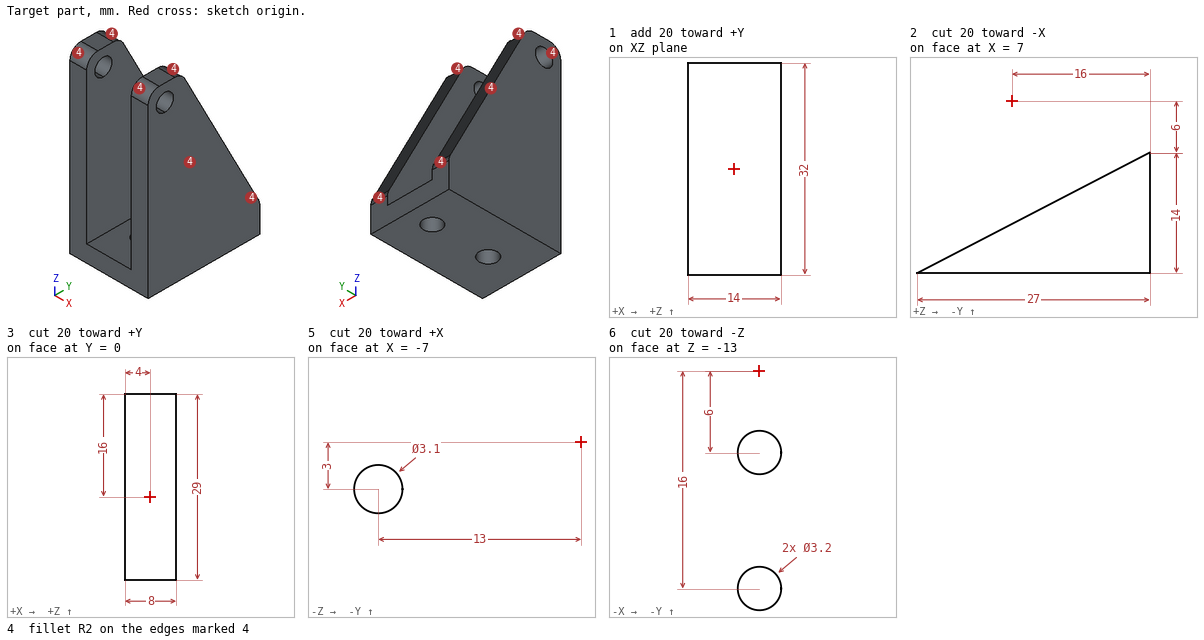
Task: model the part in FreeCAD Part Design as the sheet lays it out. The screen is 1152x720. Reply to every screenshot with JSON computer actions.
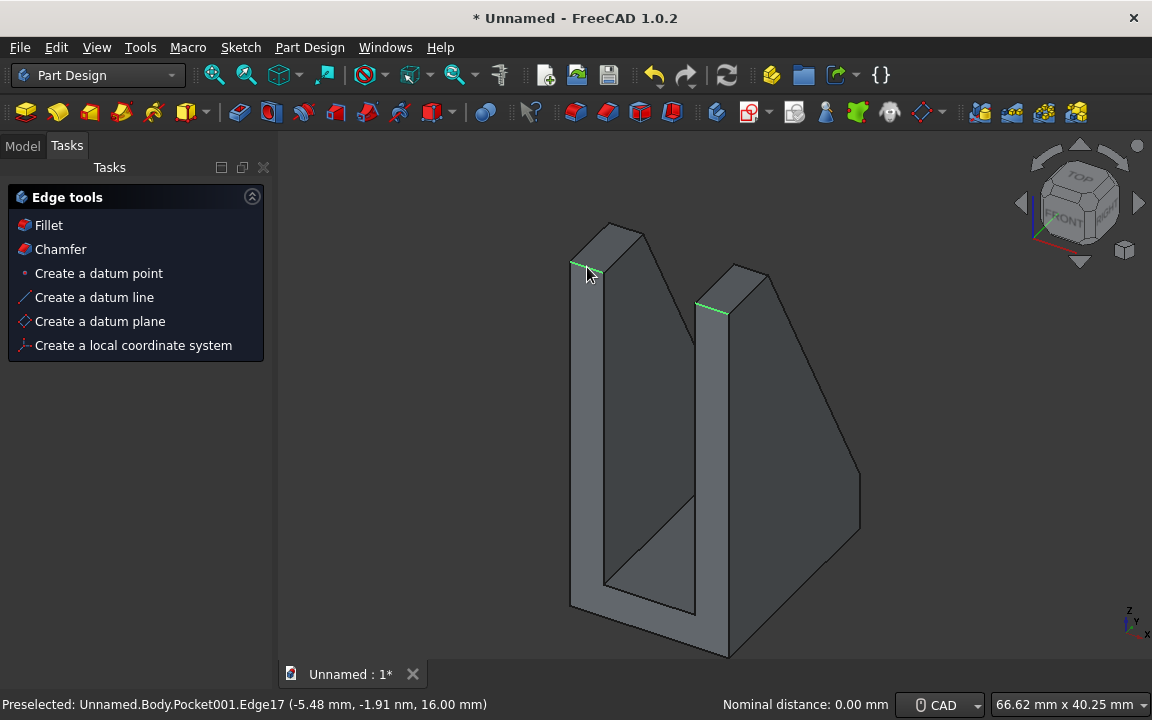
{"action": "key", "text": "0"}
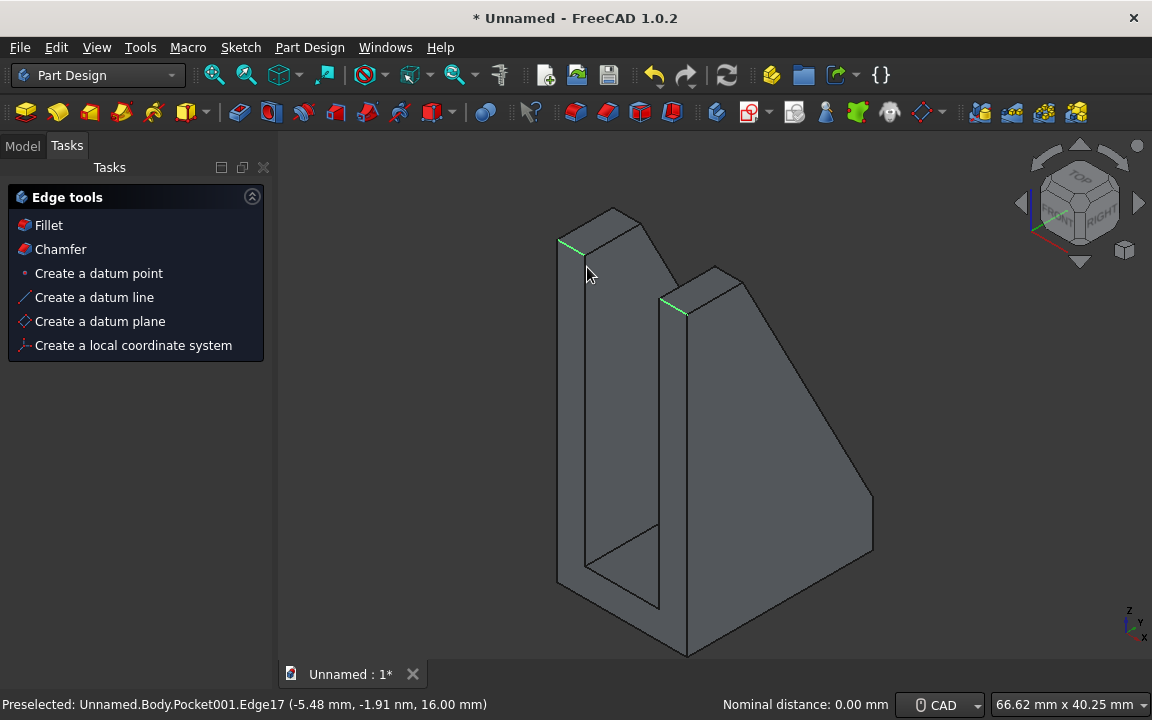
{"action": "key", "text": "2"}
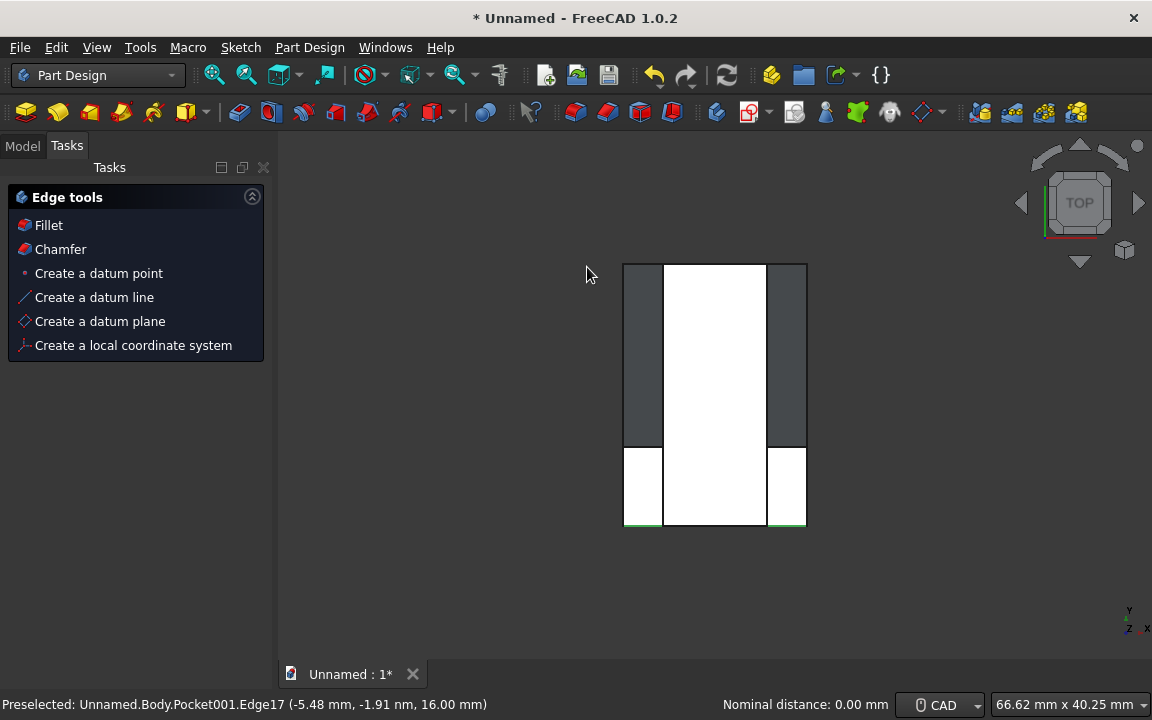
{"action": "left_click", "coordinate": [643, 446], "text": "ctrl"}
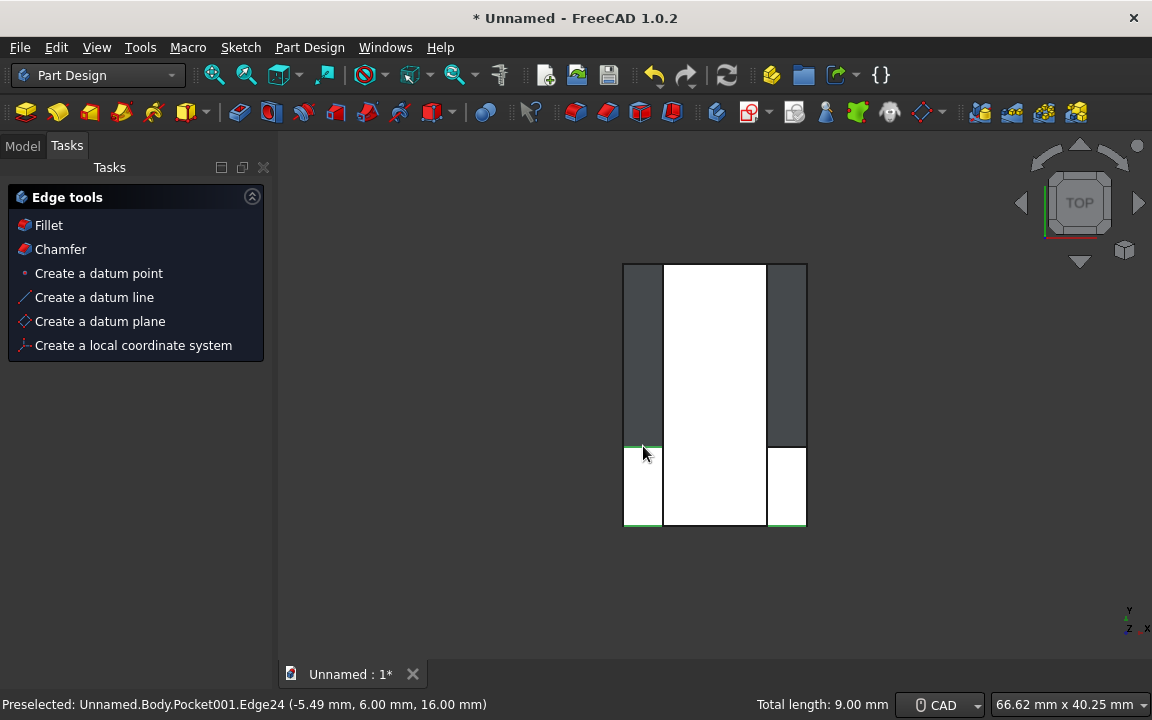
{"action": "left_click", "coordinate": [787, 446], "text": "ctrl"}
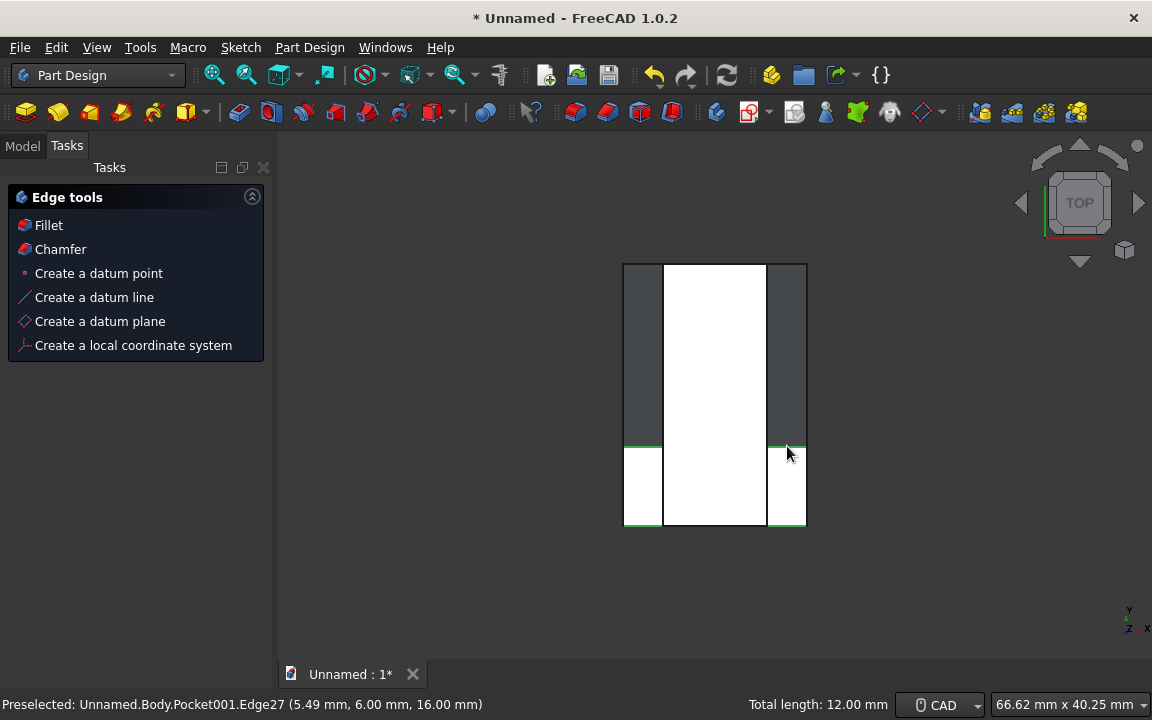
{"action": "key", "text": "1"}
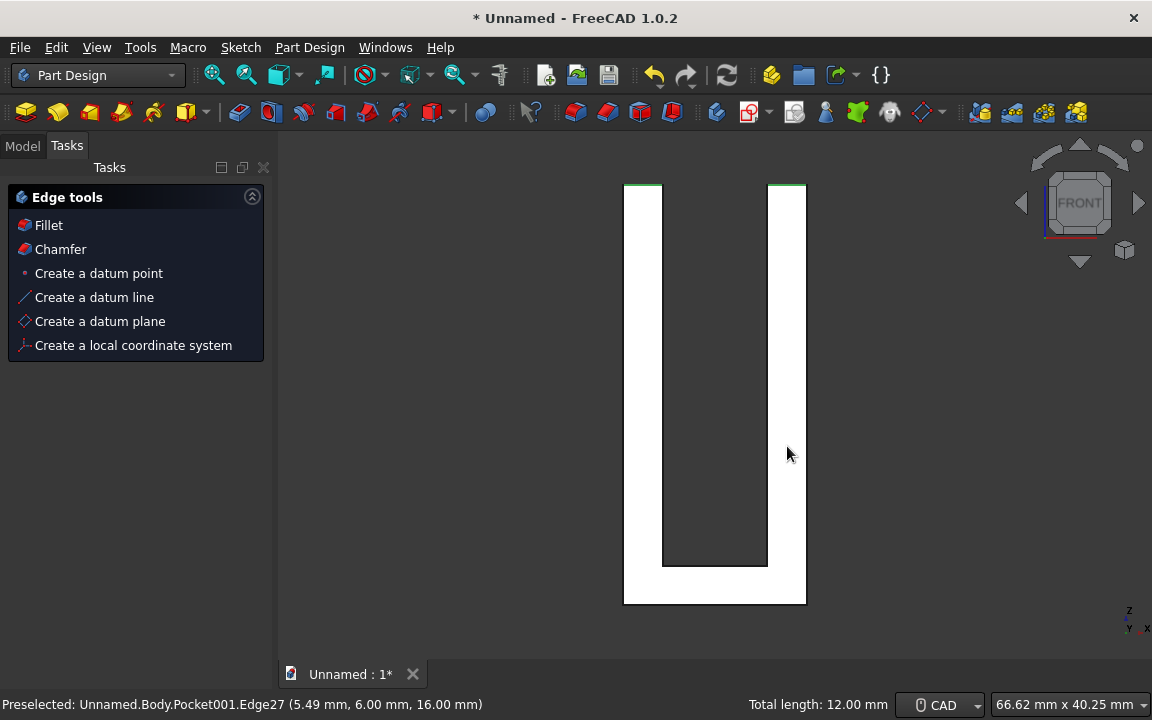
{"action": "key", "text": "3"}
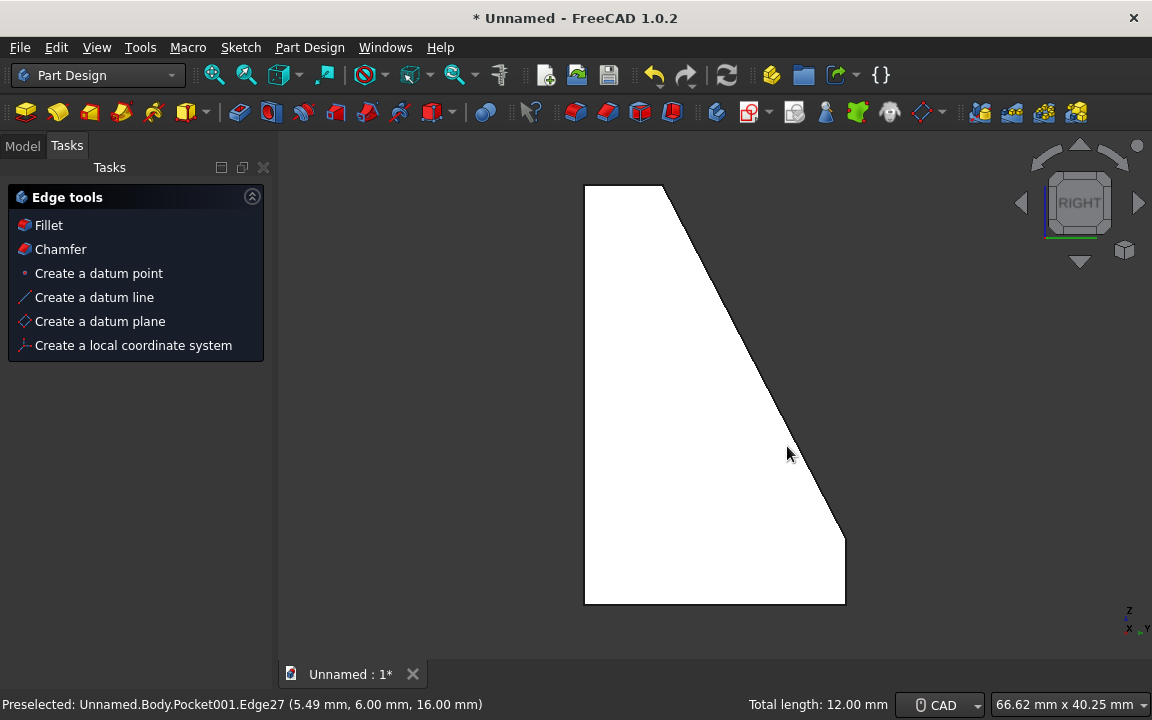
{"action": "key", "text": "5"}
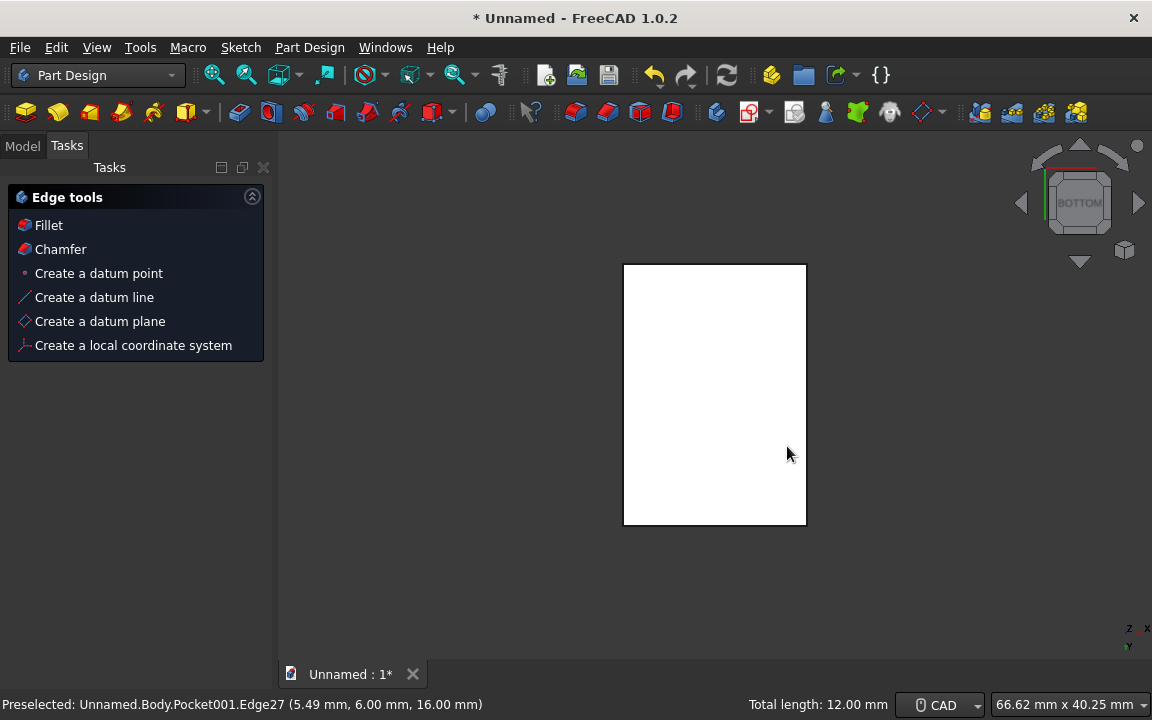
{"action": "key", "text": "4"}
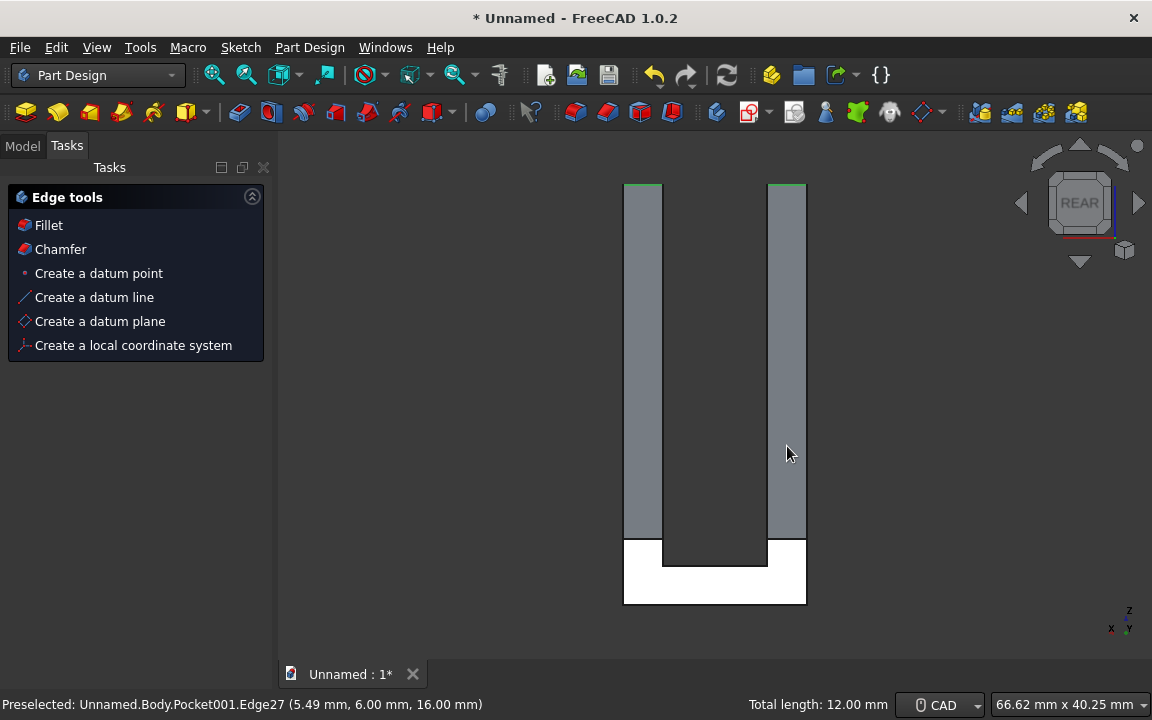
{"action": "key", "text": "6"}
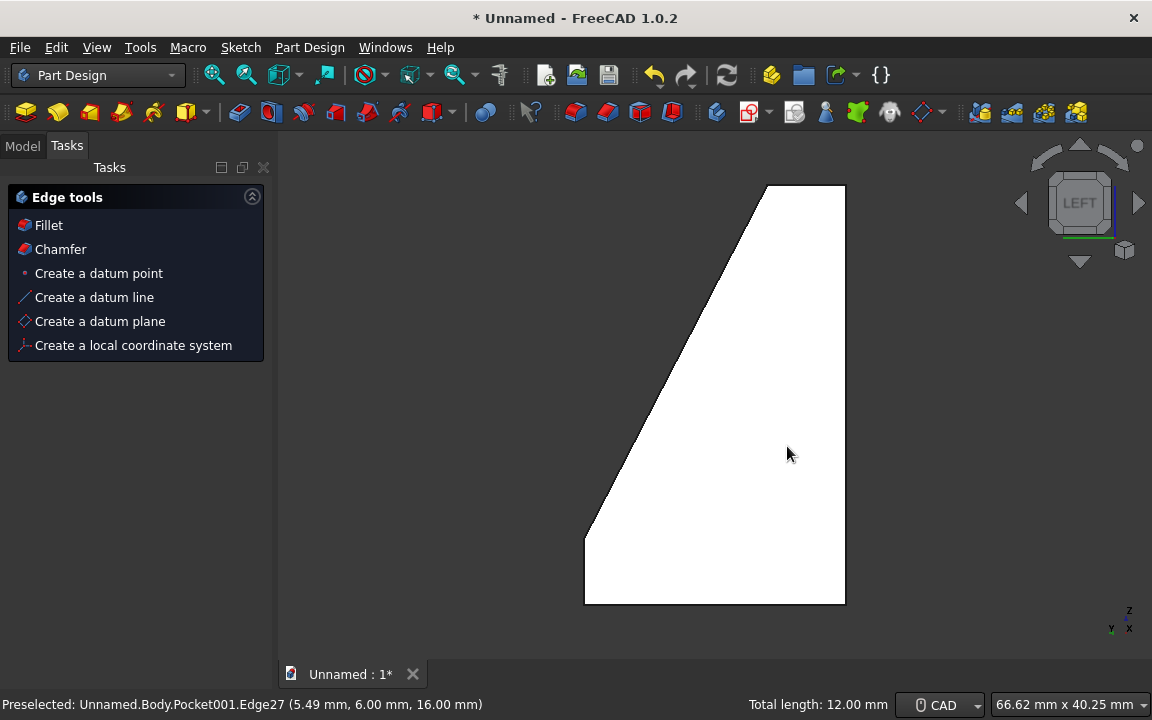
{"action": "key", "text": "v 3"}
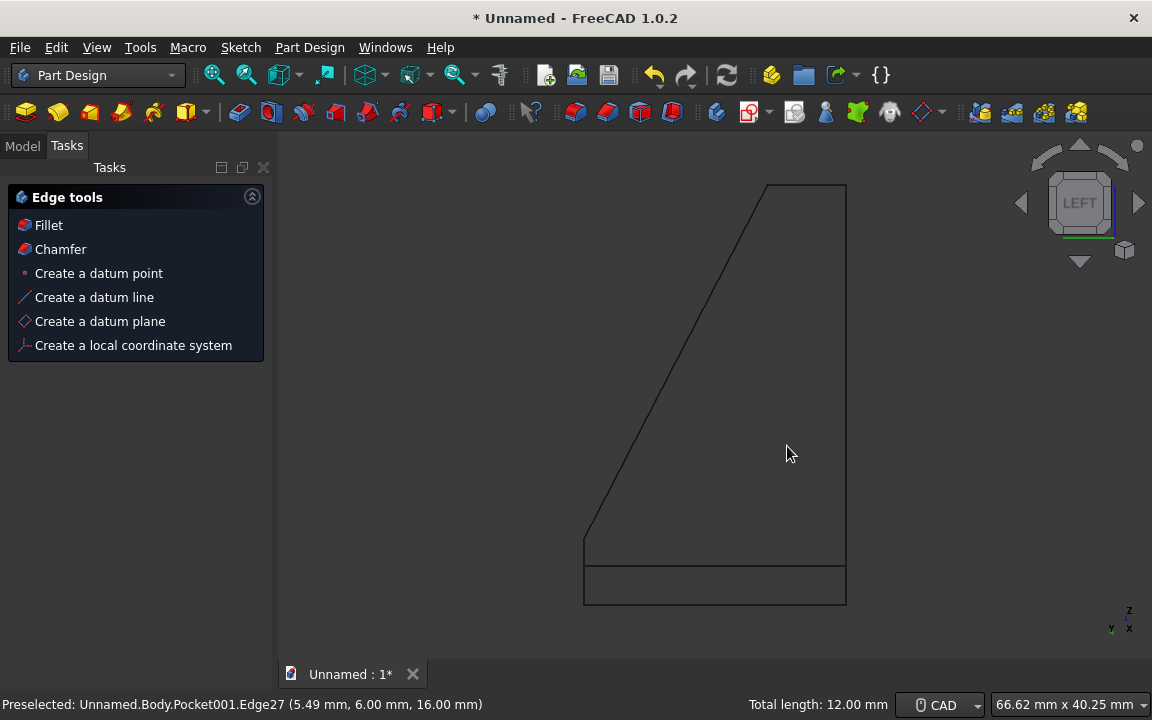
{"action": "key", "text": "0"}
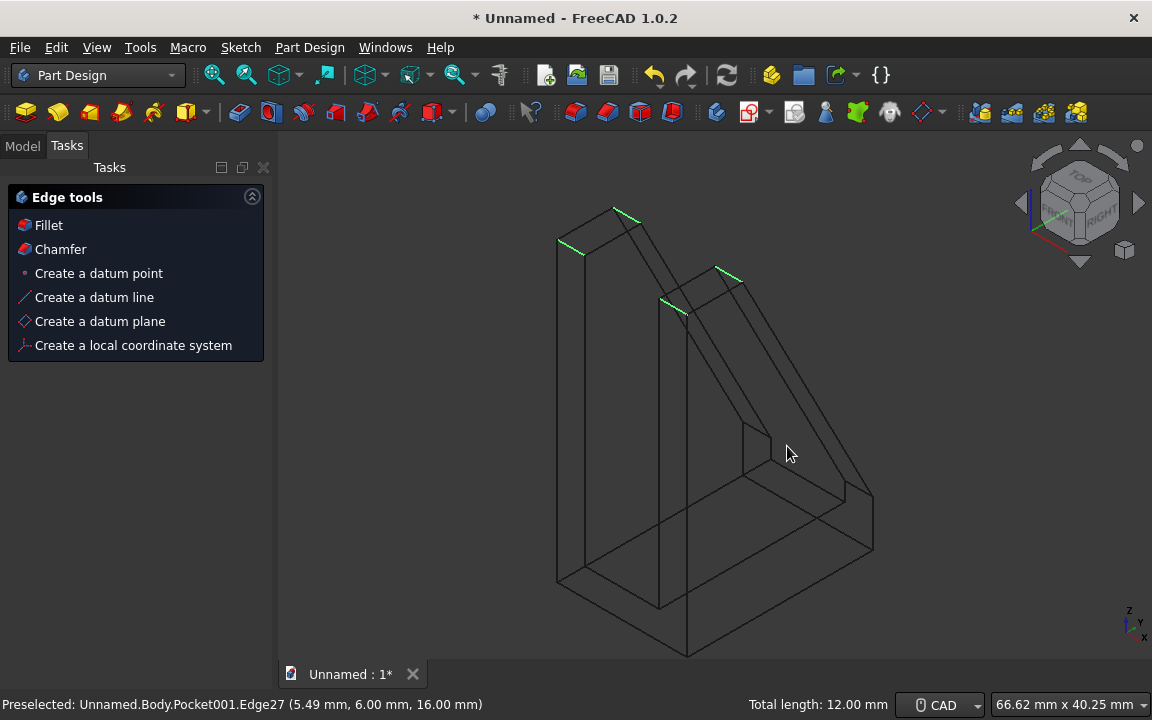
{"action": "left_click", "coordinate": [757, 429], "text": "ctrl"}